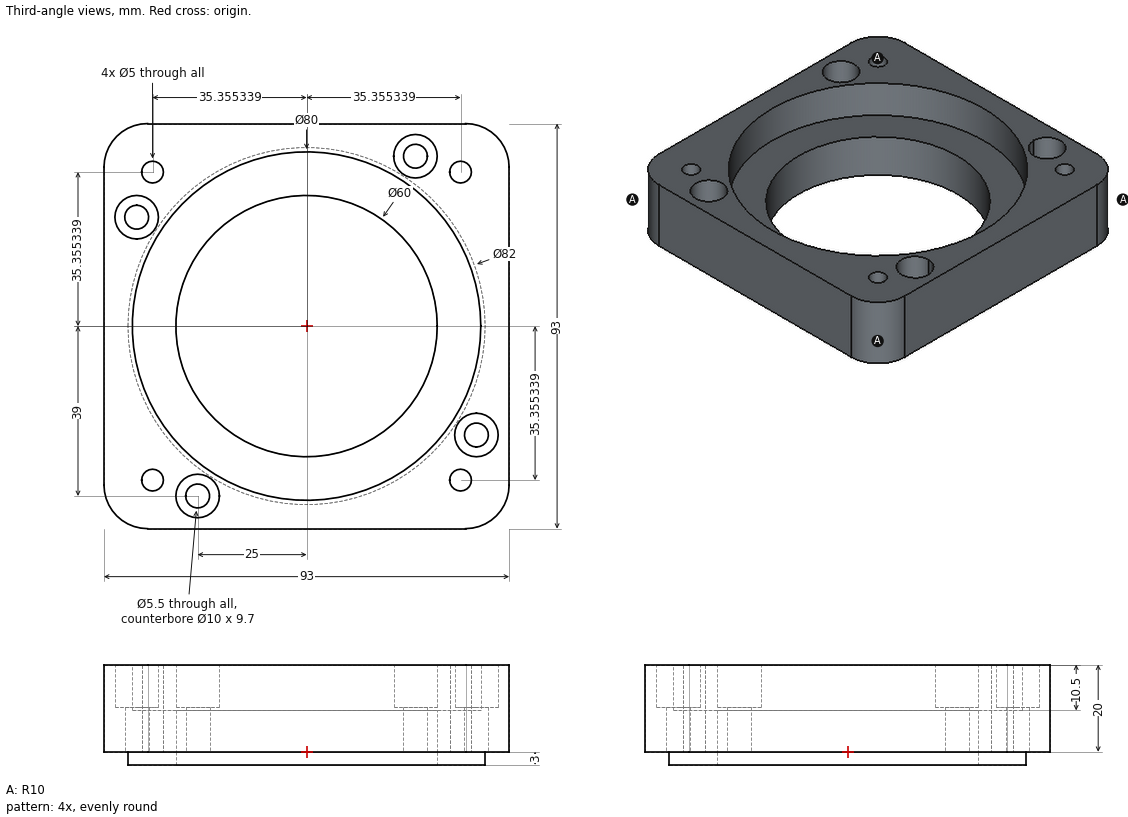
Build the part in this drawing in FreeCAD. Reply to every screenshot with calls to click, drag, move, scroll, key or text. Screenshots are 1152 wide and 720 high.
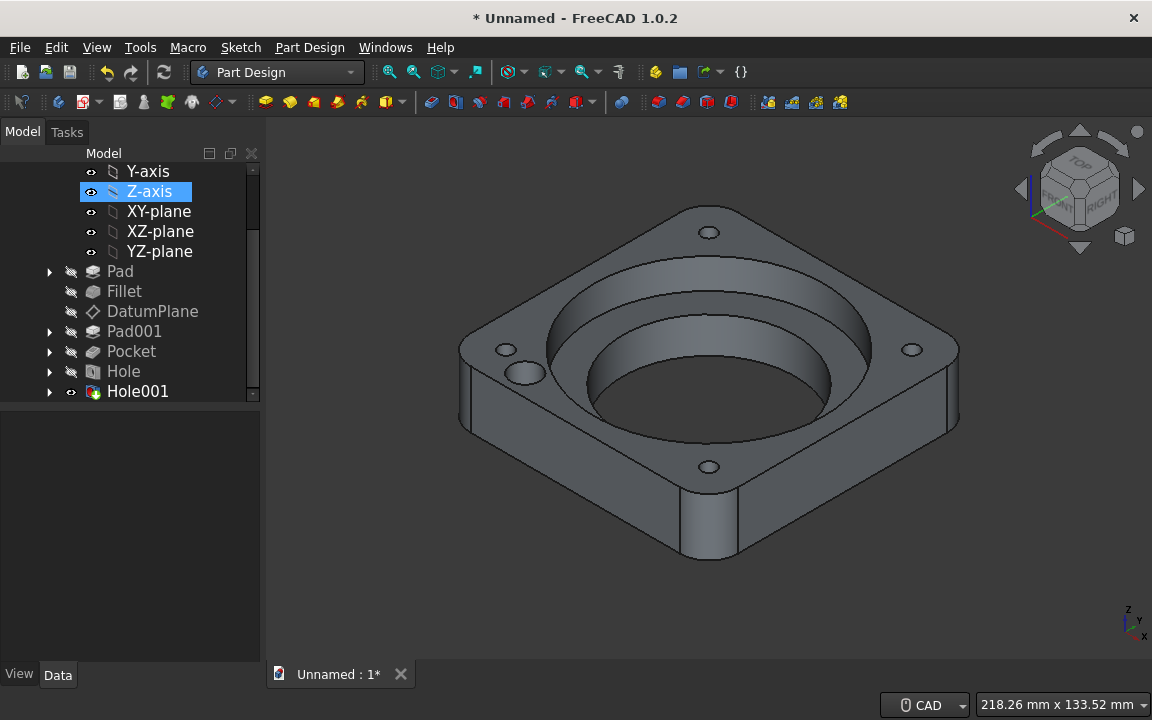
click(116, 392)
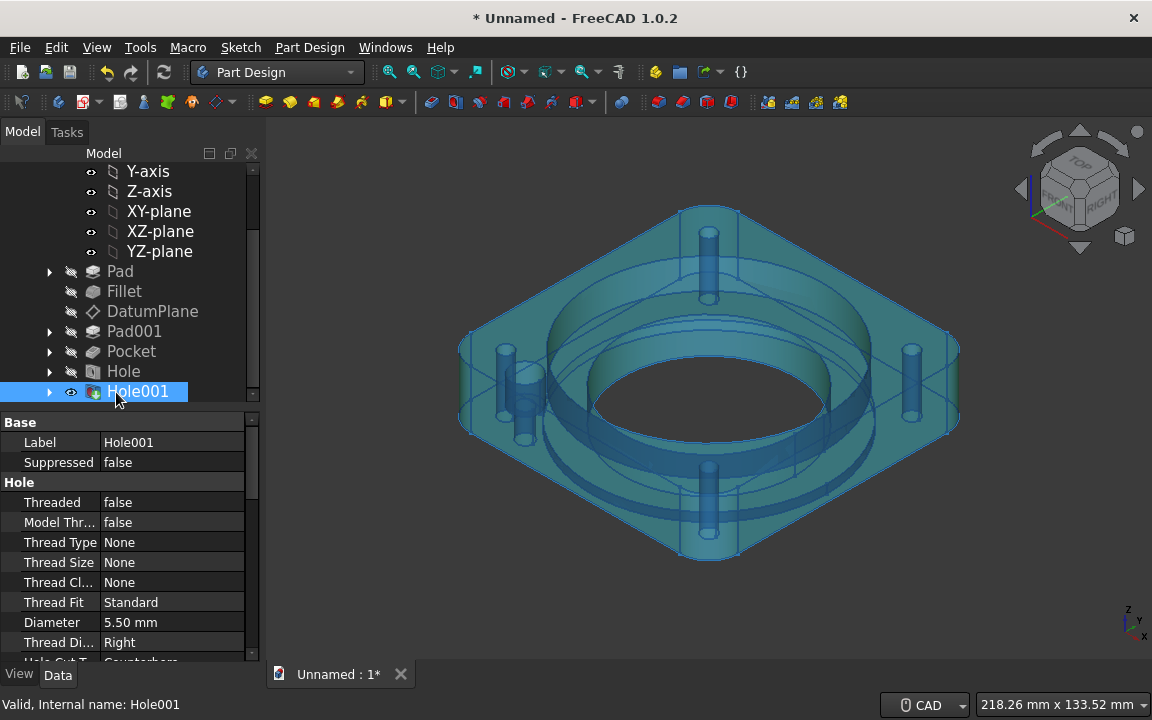
click(816, 102)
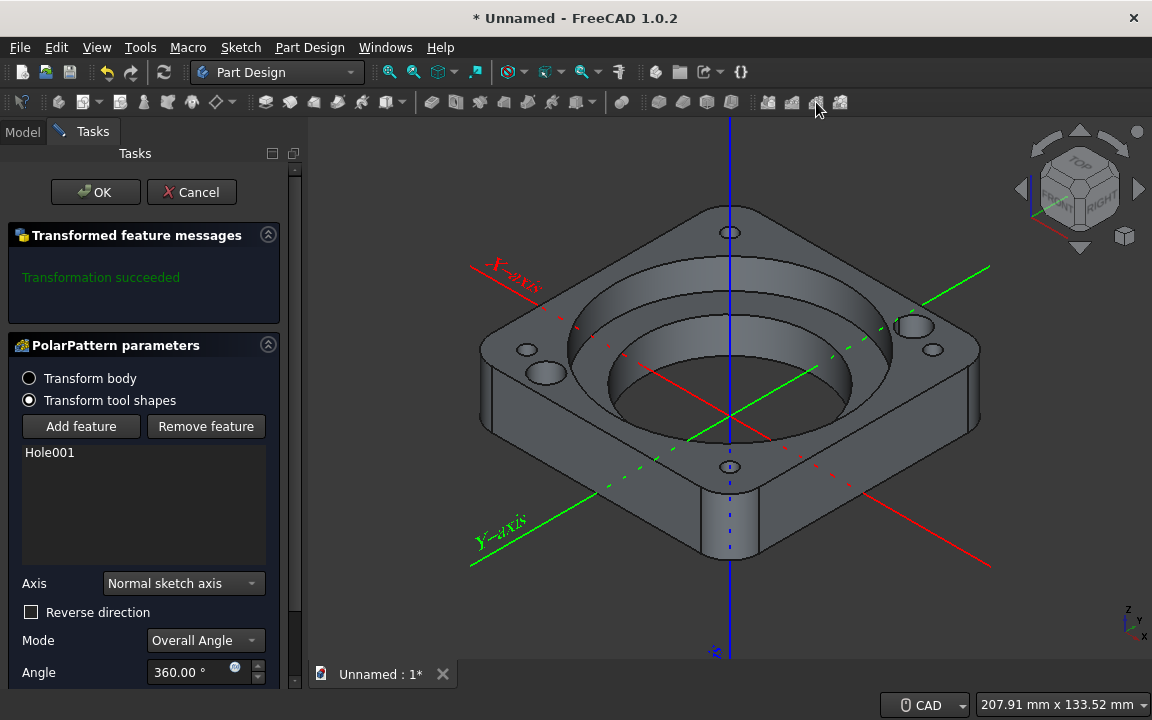
click(184, 584)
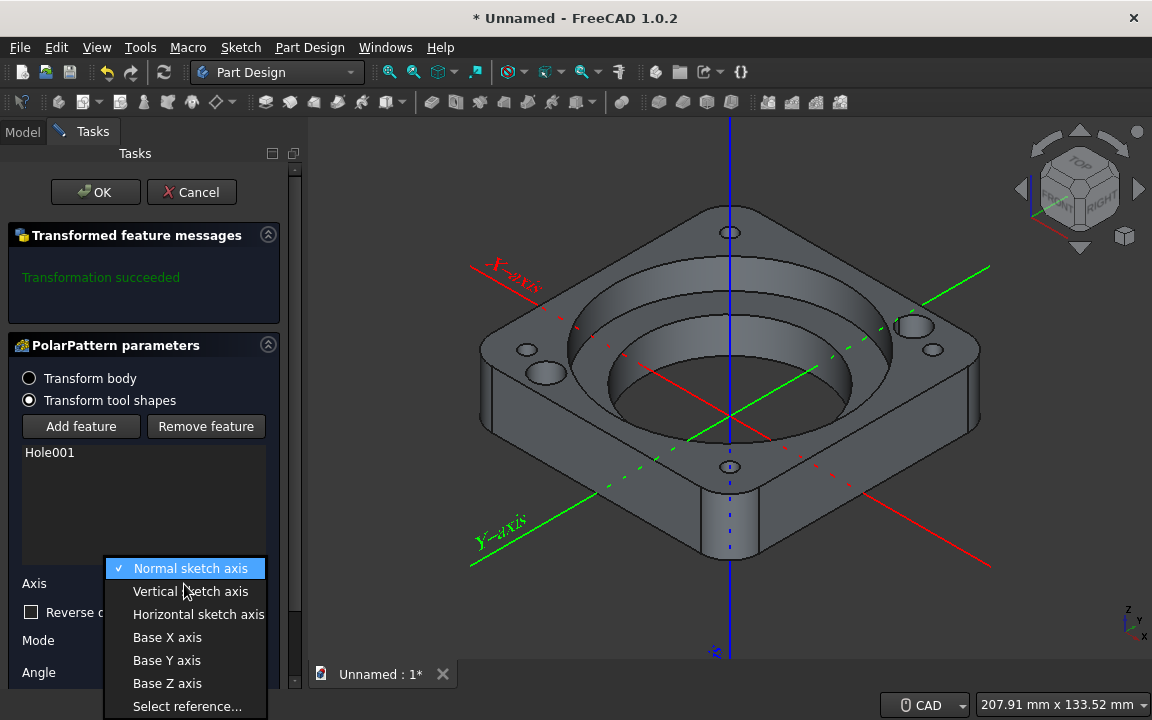
click(184, 684)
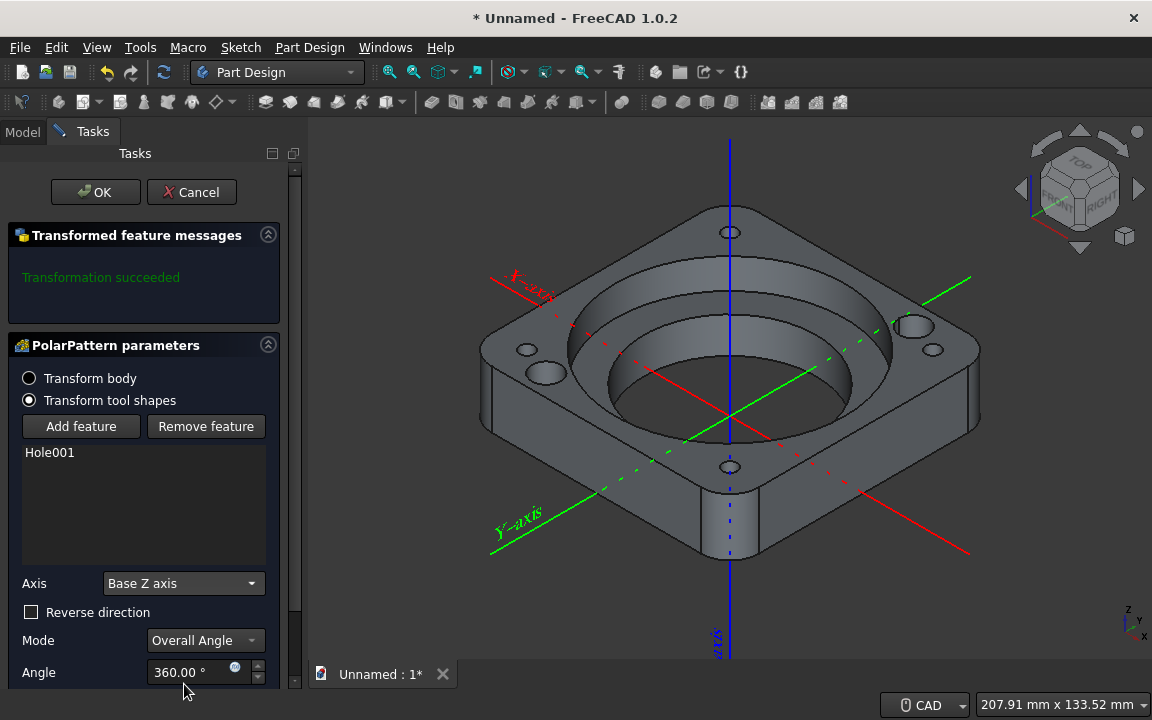
scroll(295, 426, down, 2)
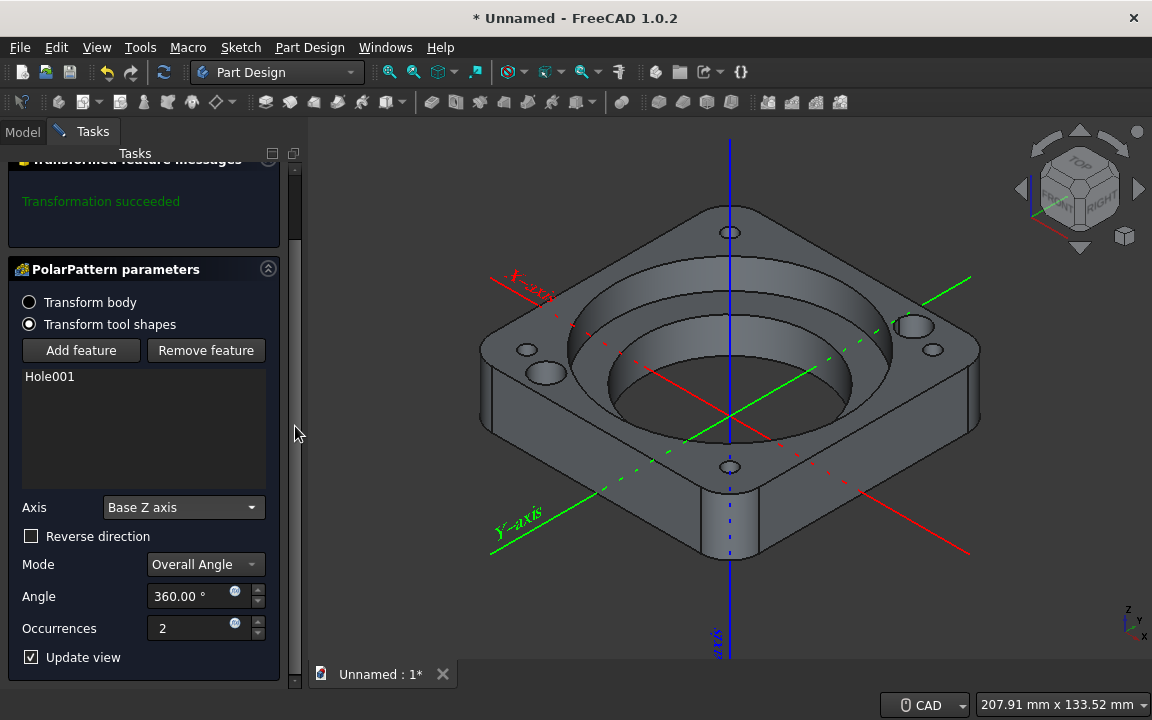
triple_click(198, 628)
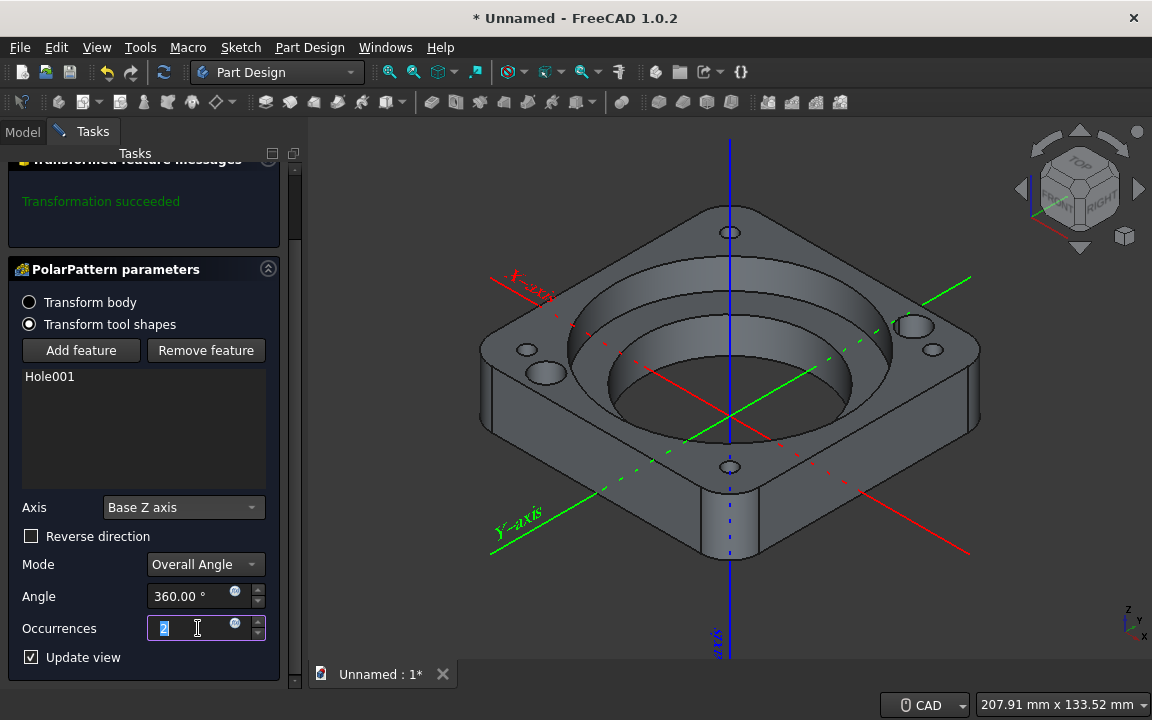
text(4)
key(Tab)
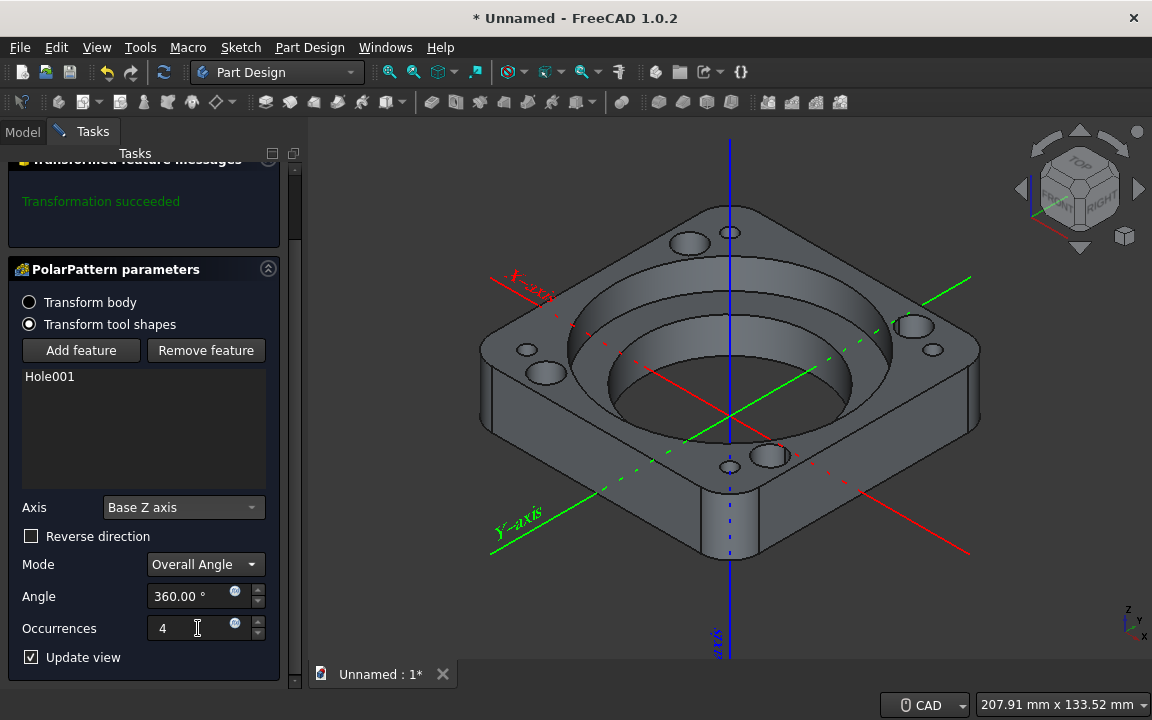
scroll(295, 426, up, 3)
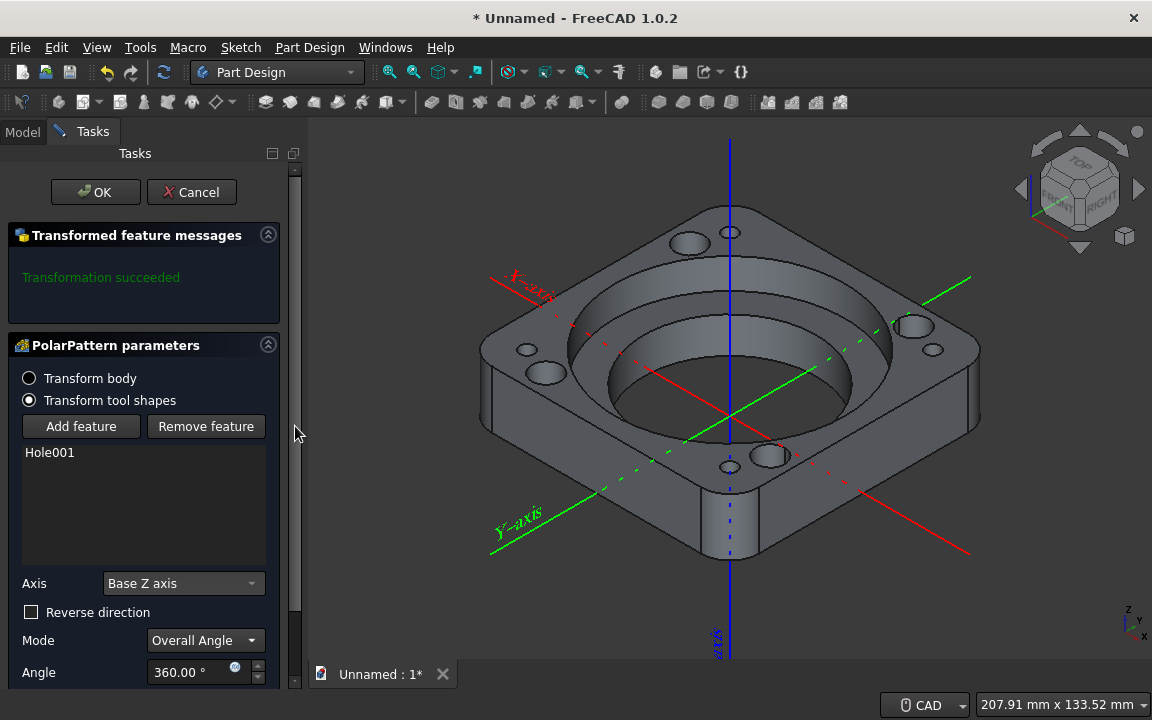
click(96, 192)